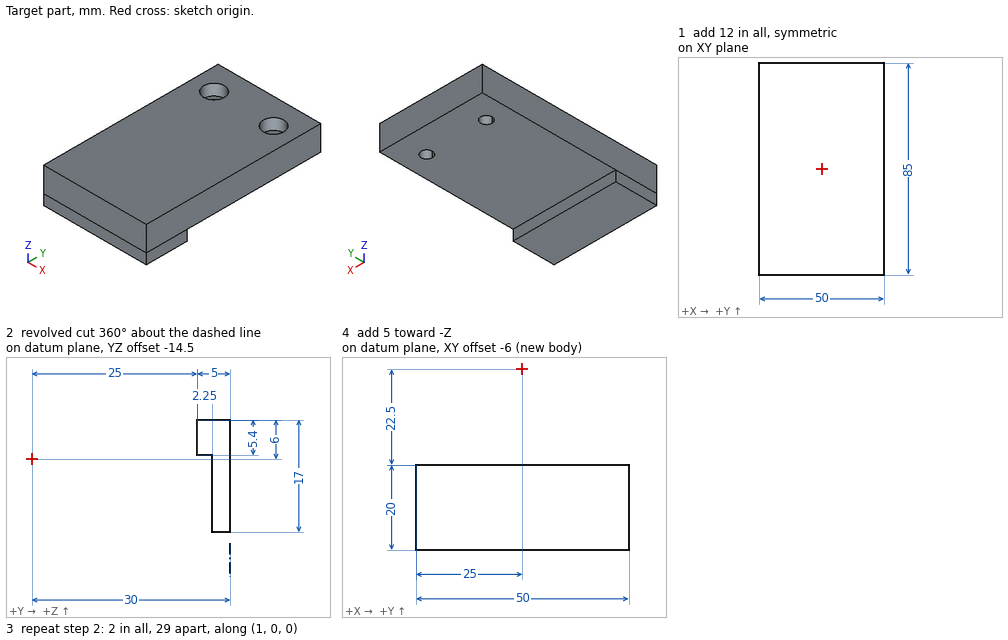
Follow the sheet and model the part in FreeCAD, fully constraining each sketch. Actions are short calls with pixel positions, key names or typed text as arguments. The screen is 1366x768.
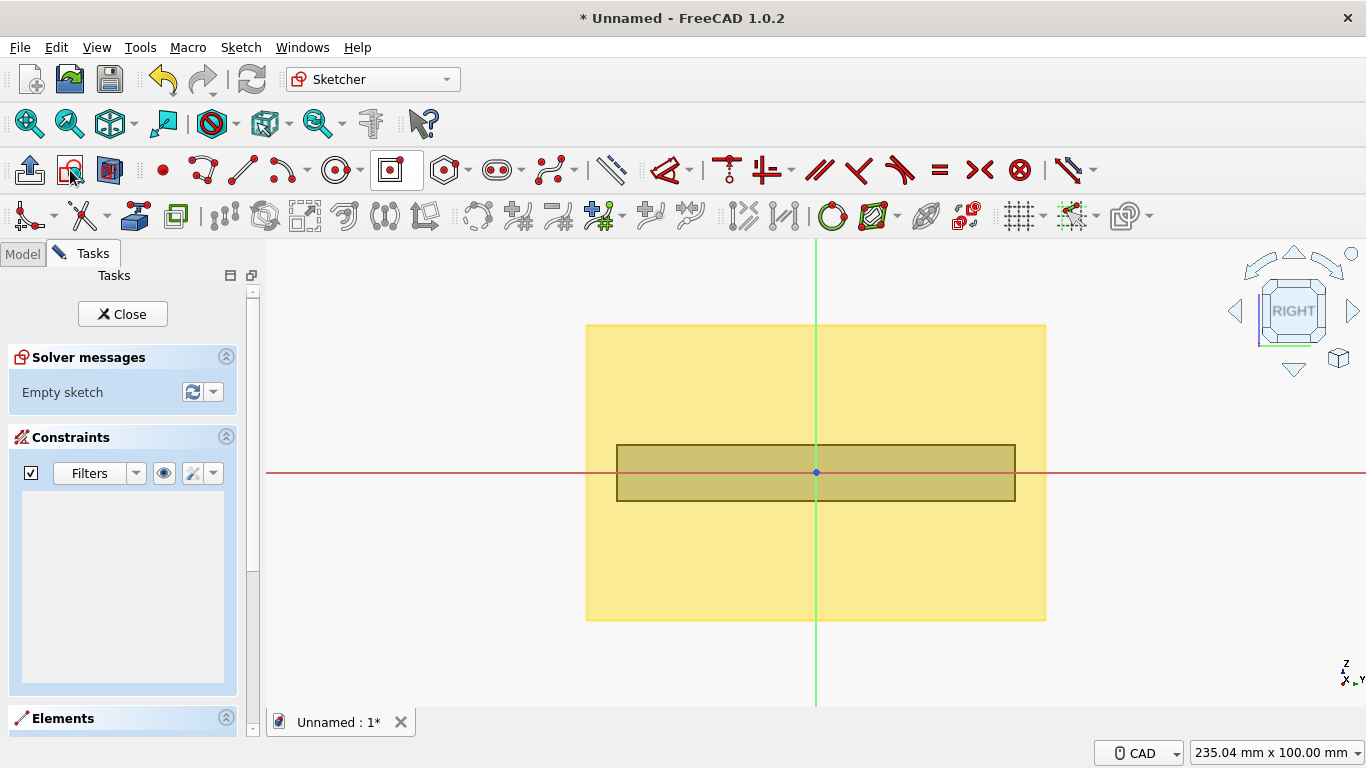
scroll(967, 517, up, 5)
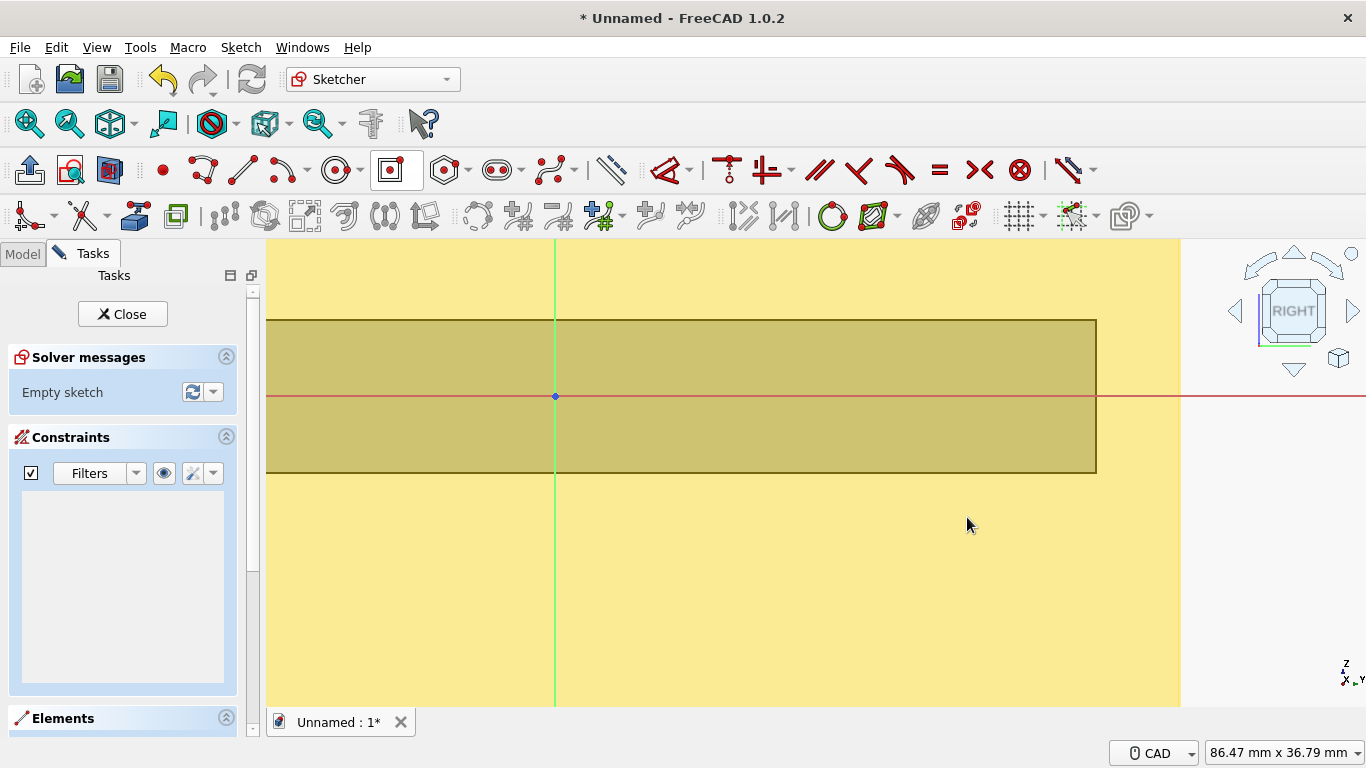
key(g)
key(m)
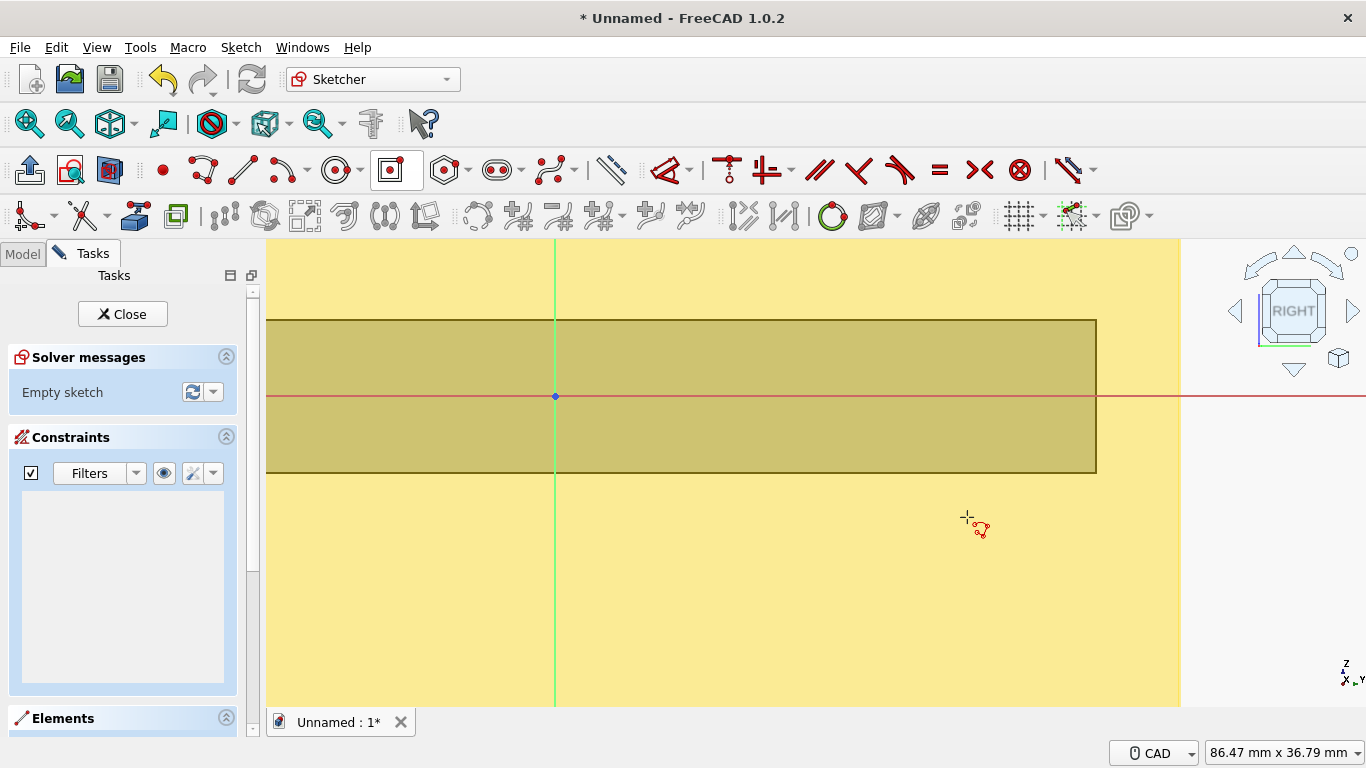
scroll(873, 389, up, 4)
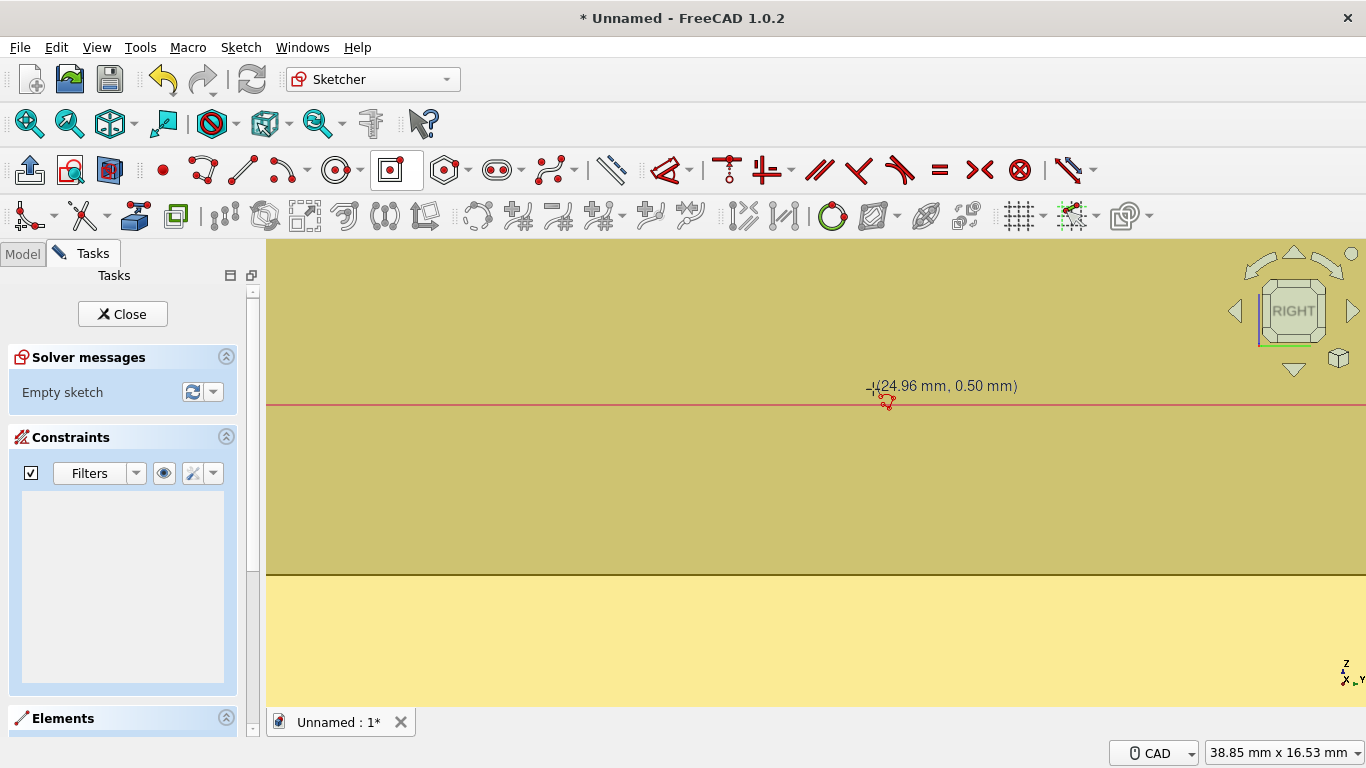
click(873, 388)
click(937, 388)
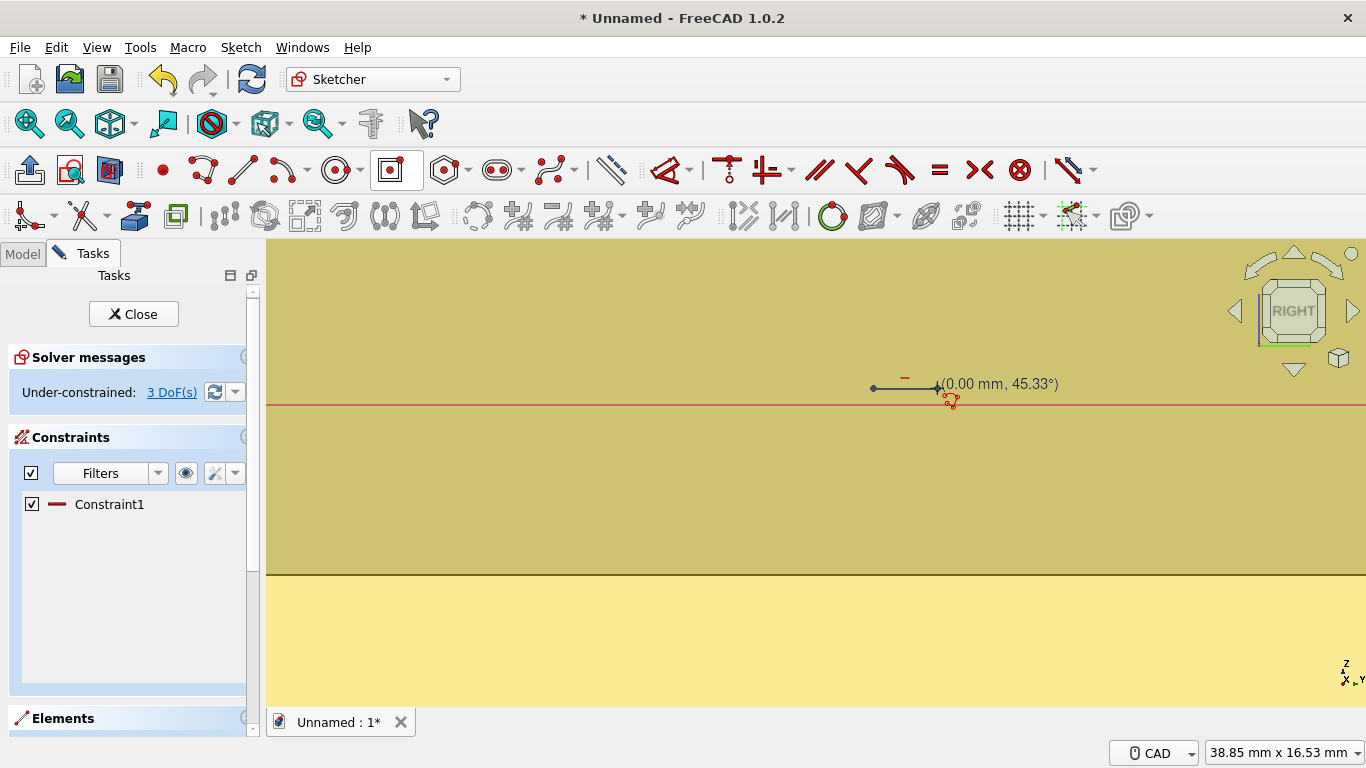
scroll(876, 392, down, 4)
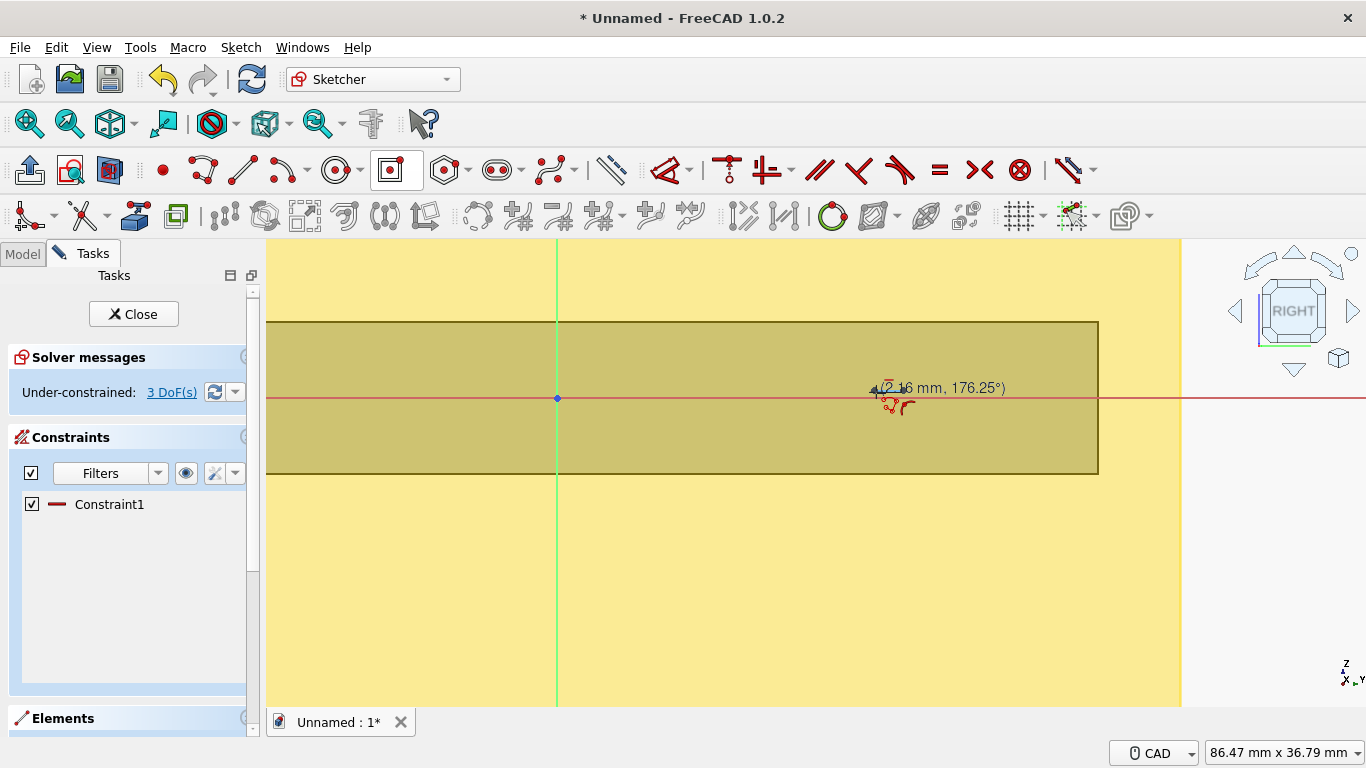
click(904, 538)
click(939, 538)
click(939, 322)
click(875, 322)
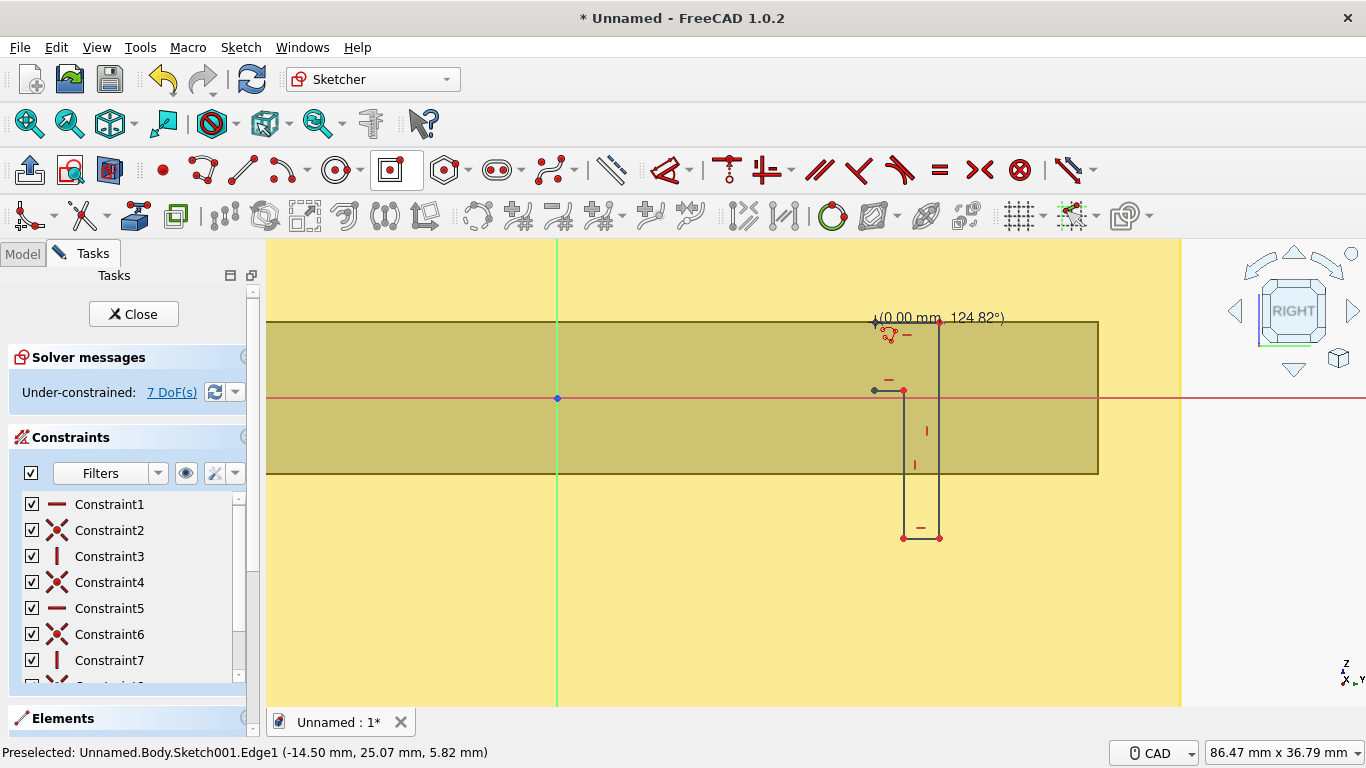
scroll(875, 390, up, 4)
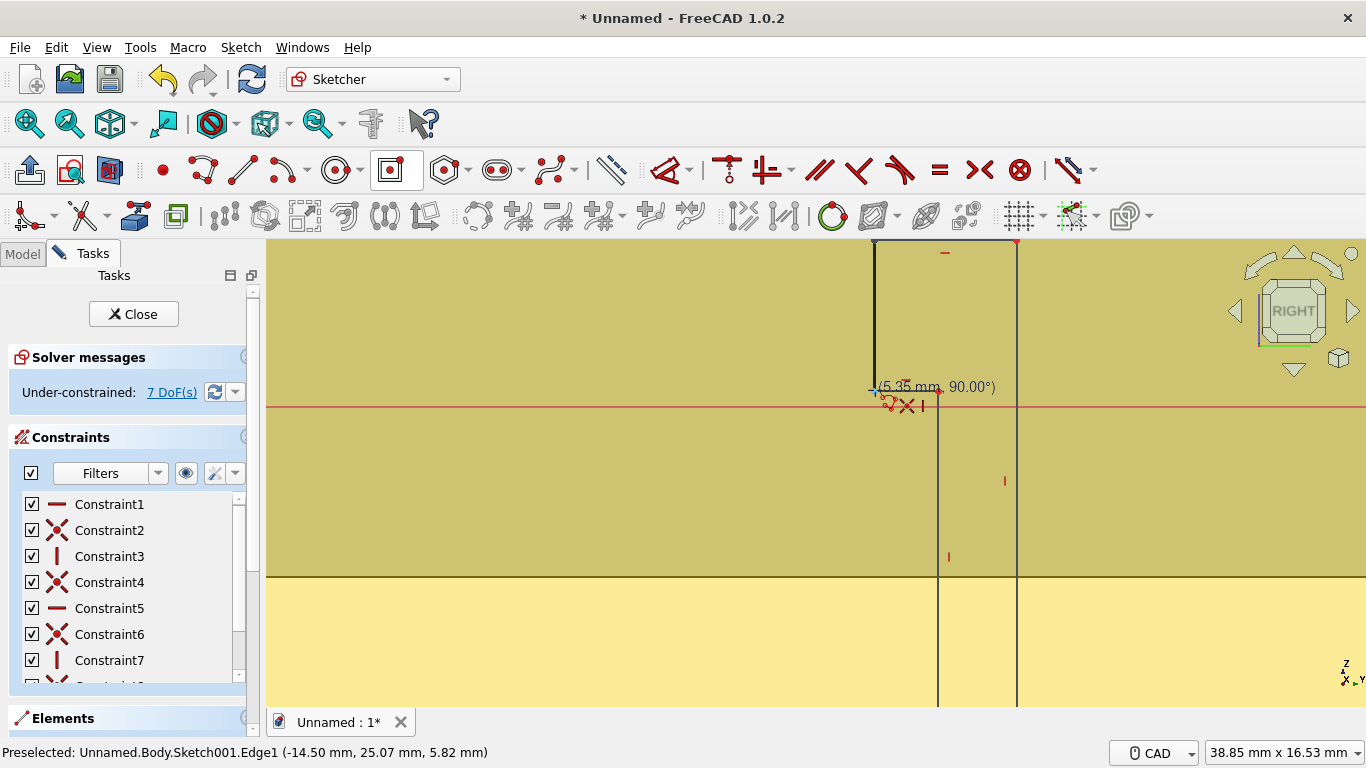
click(874, 391)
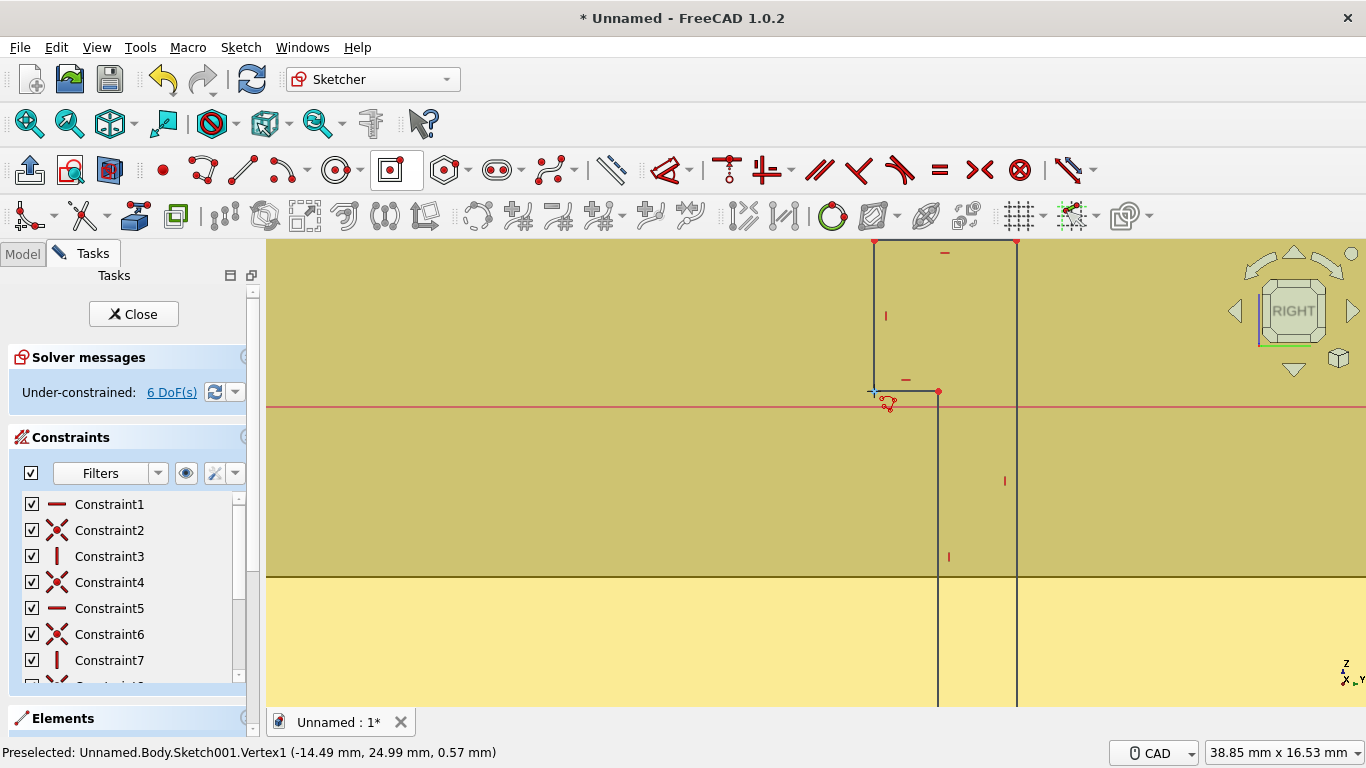
key(g)
key(l)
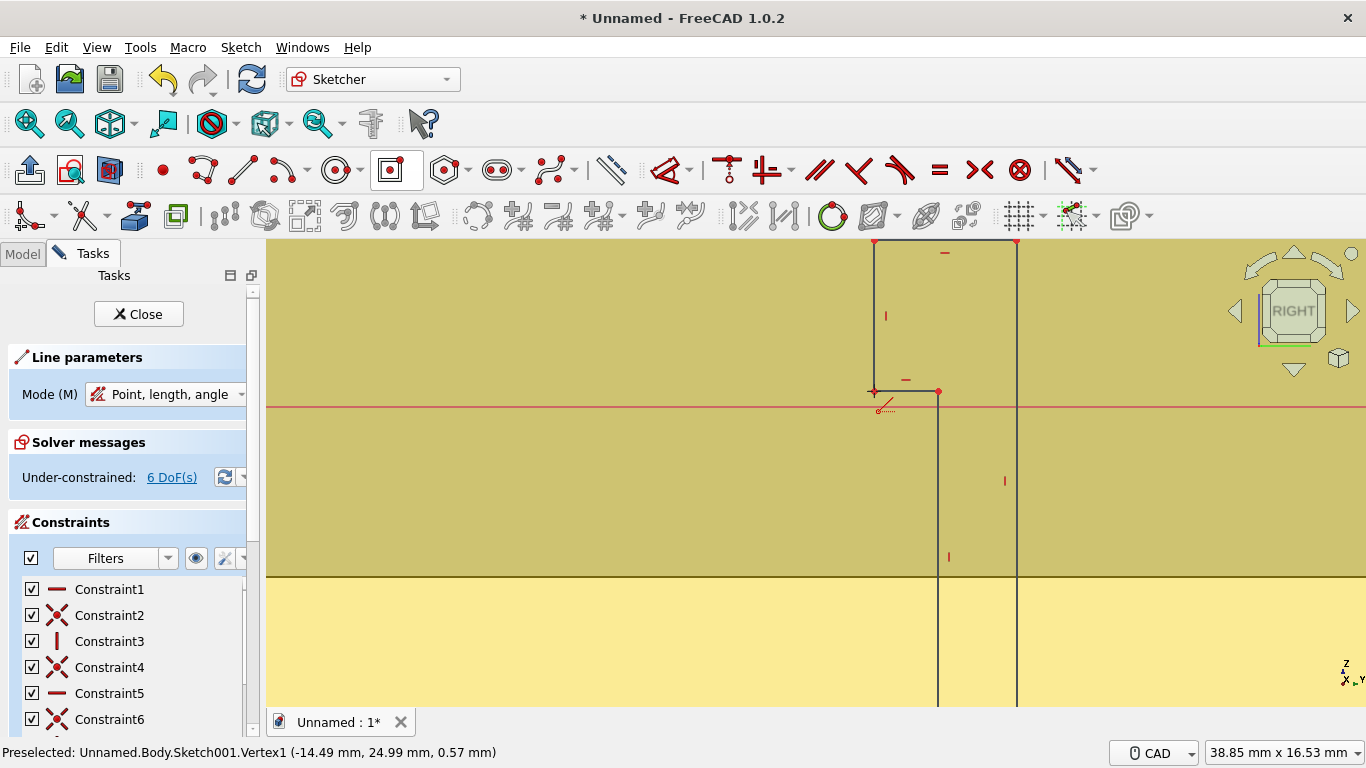
scroll(875, 390, down, 4)